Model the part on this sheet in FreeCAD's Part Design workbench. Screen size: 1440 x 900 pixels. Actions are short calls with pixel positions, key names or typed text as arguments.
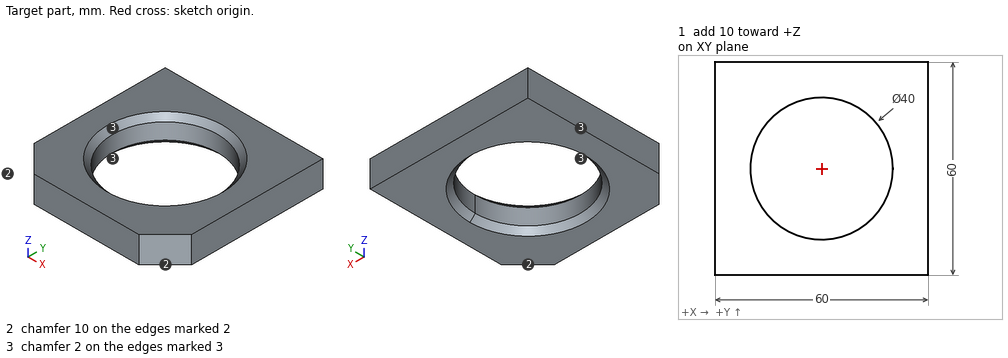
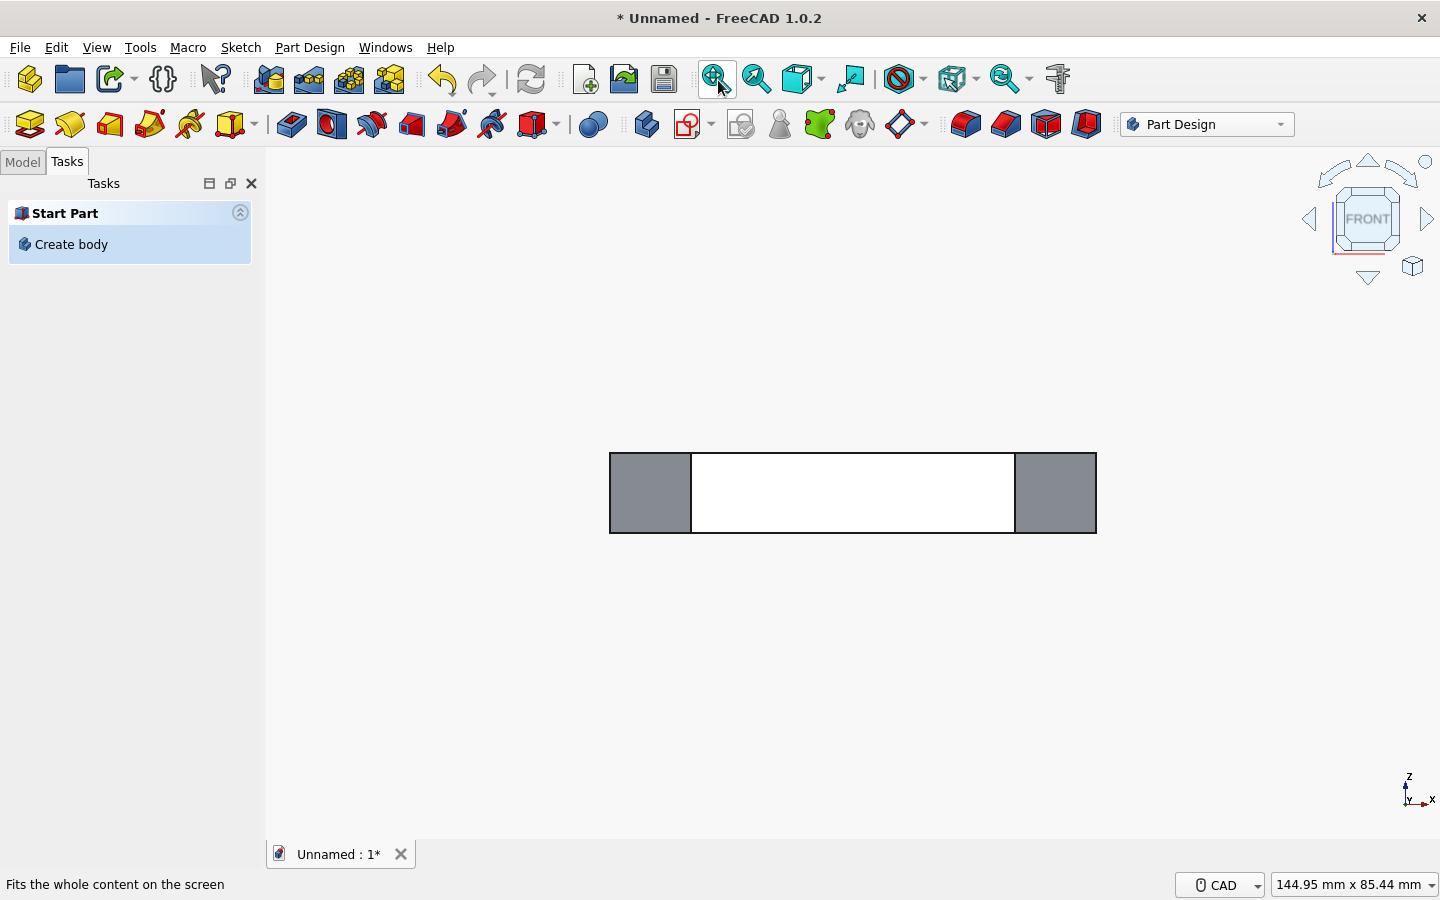
key(0)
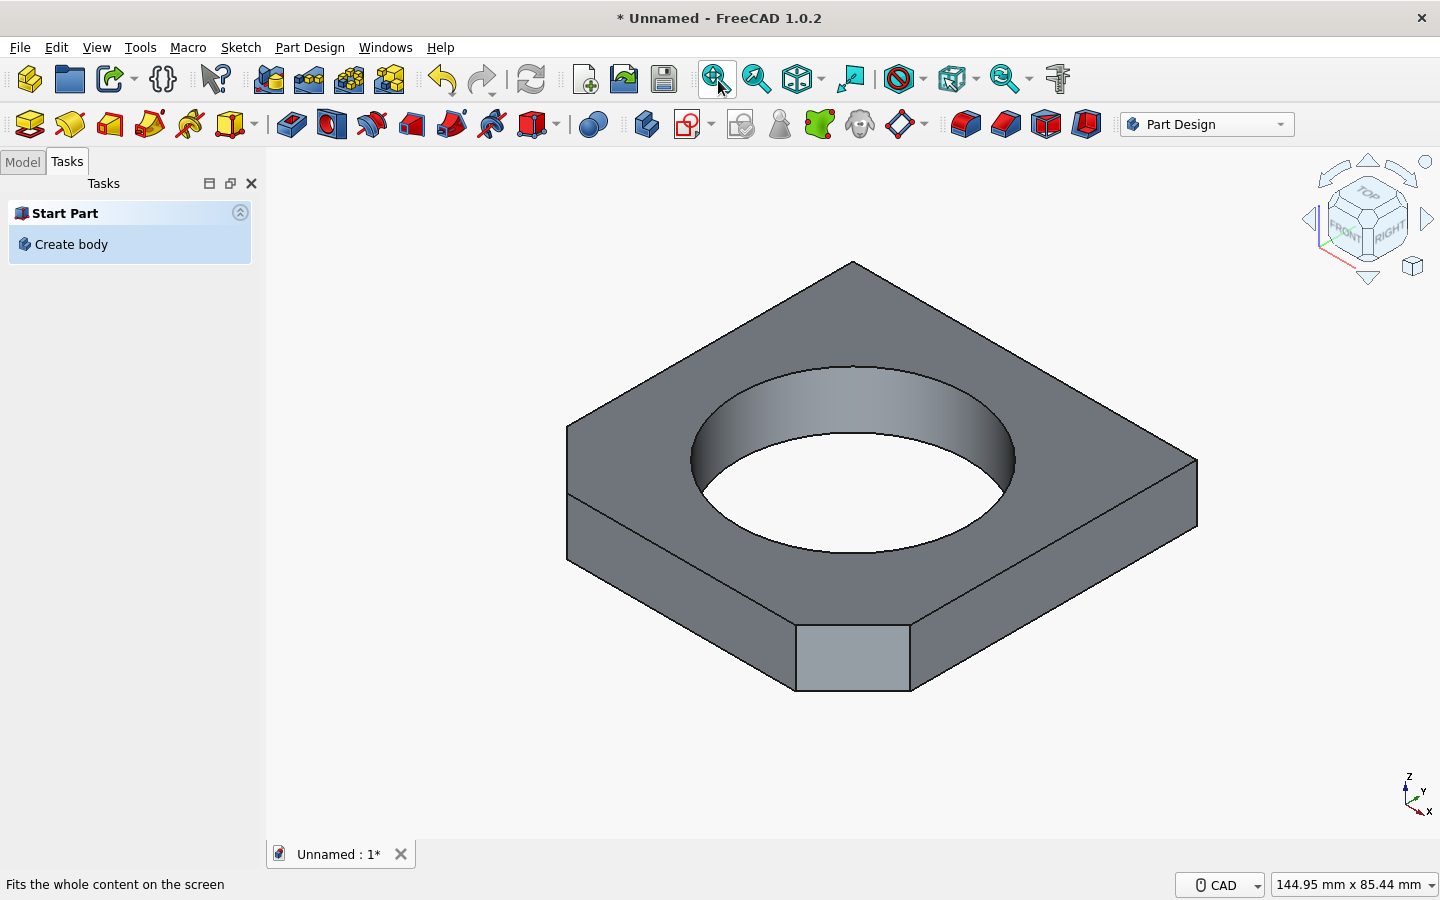
click(738, 393)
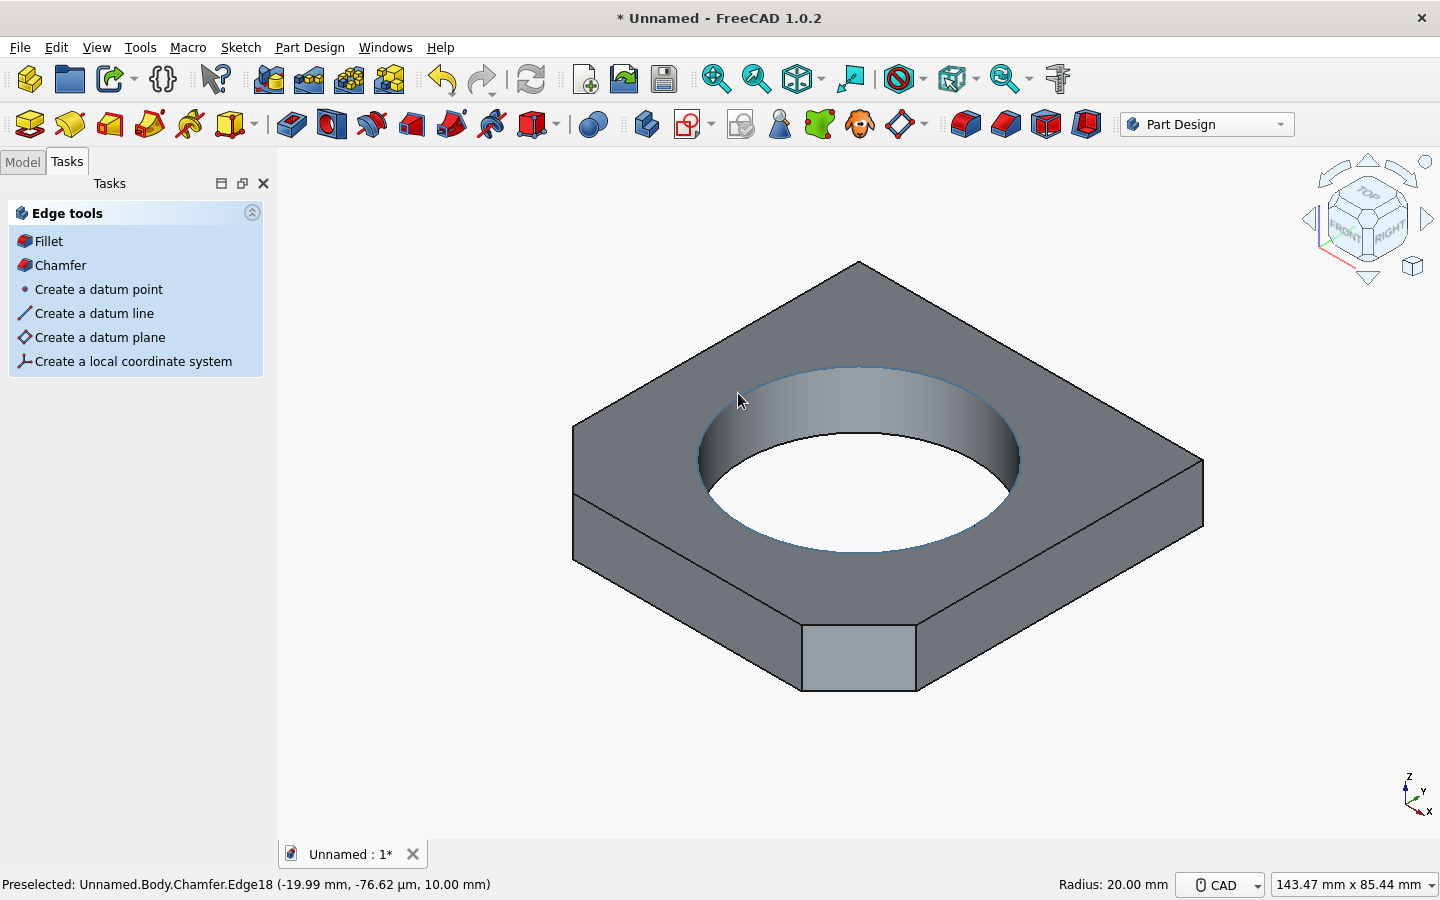
key(2)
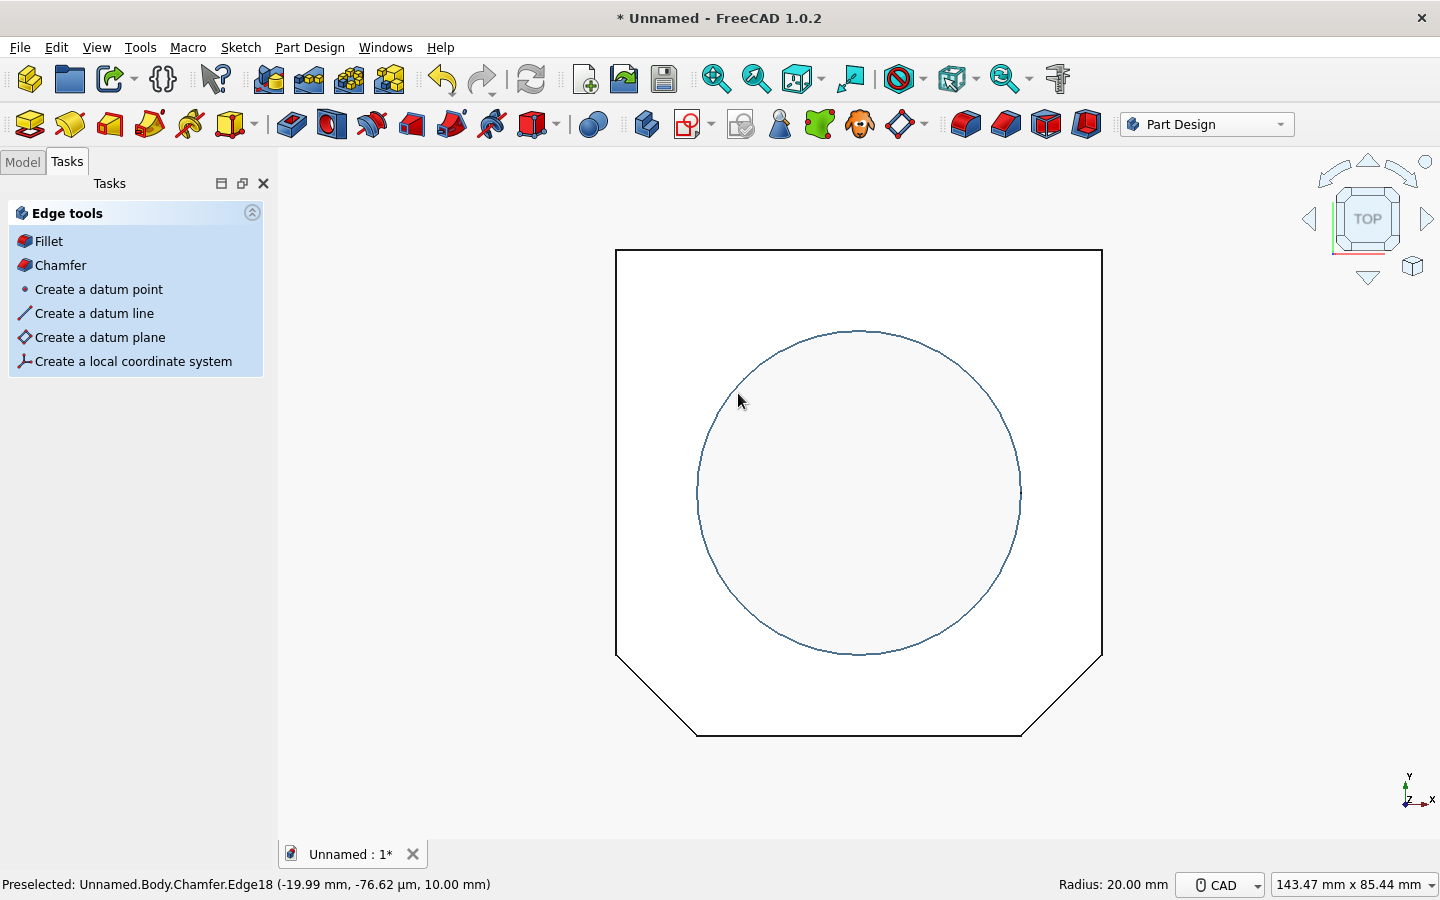
key(1)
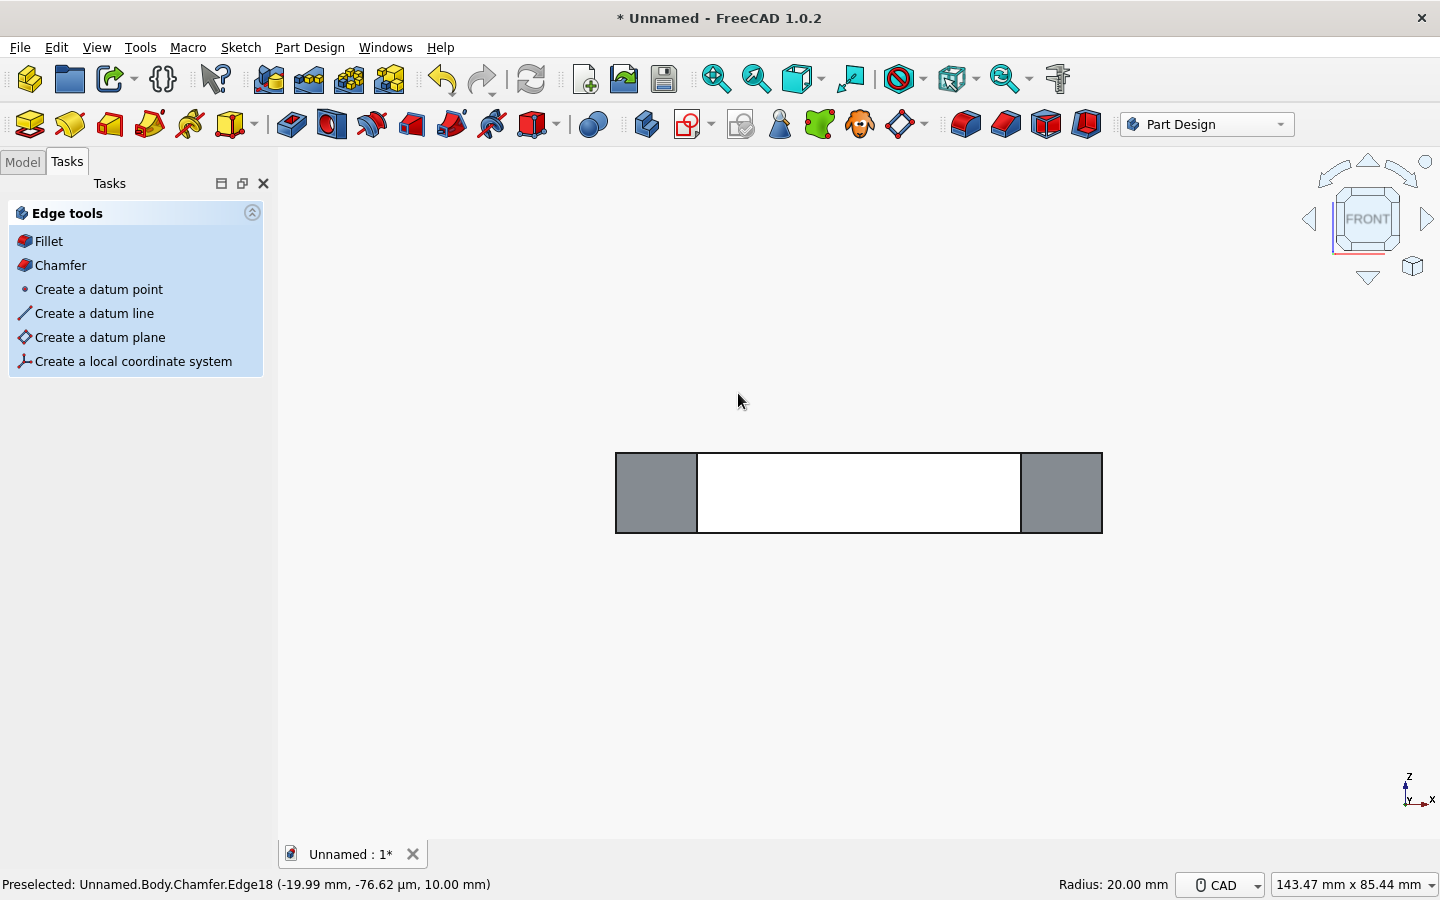
click(718, 80)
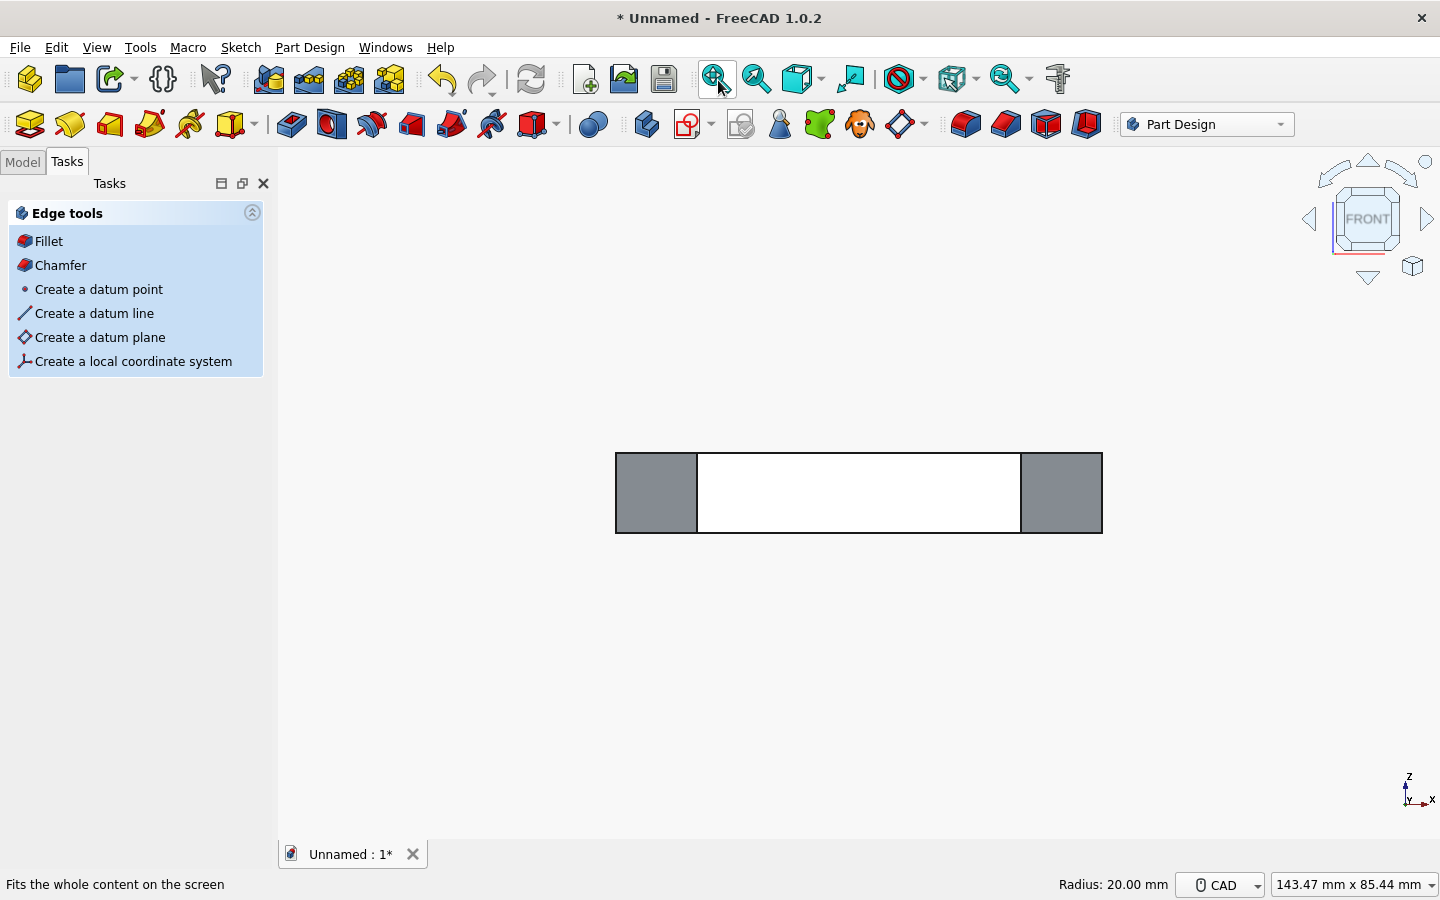
key(3)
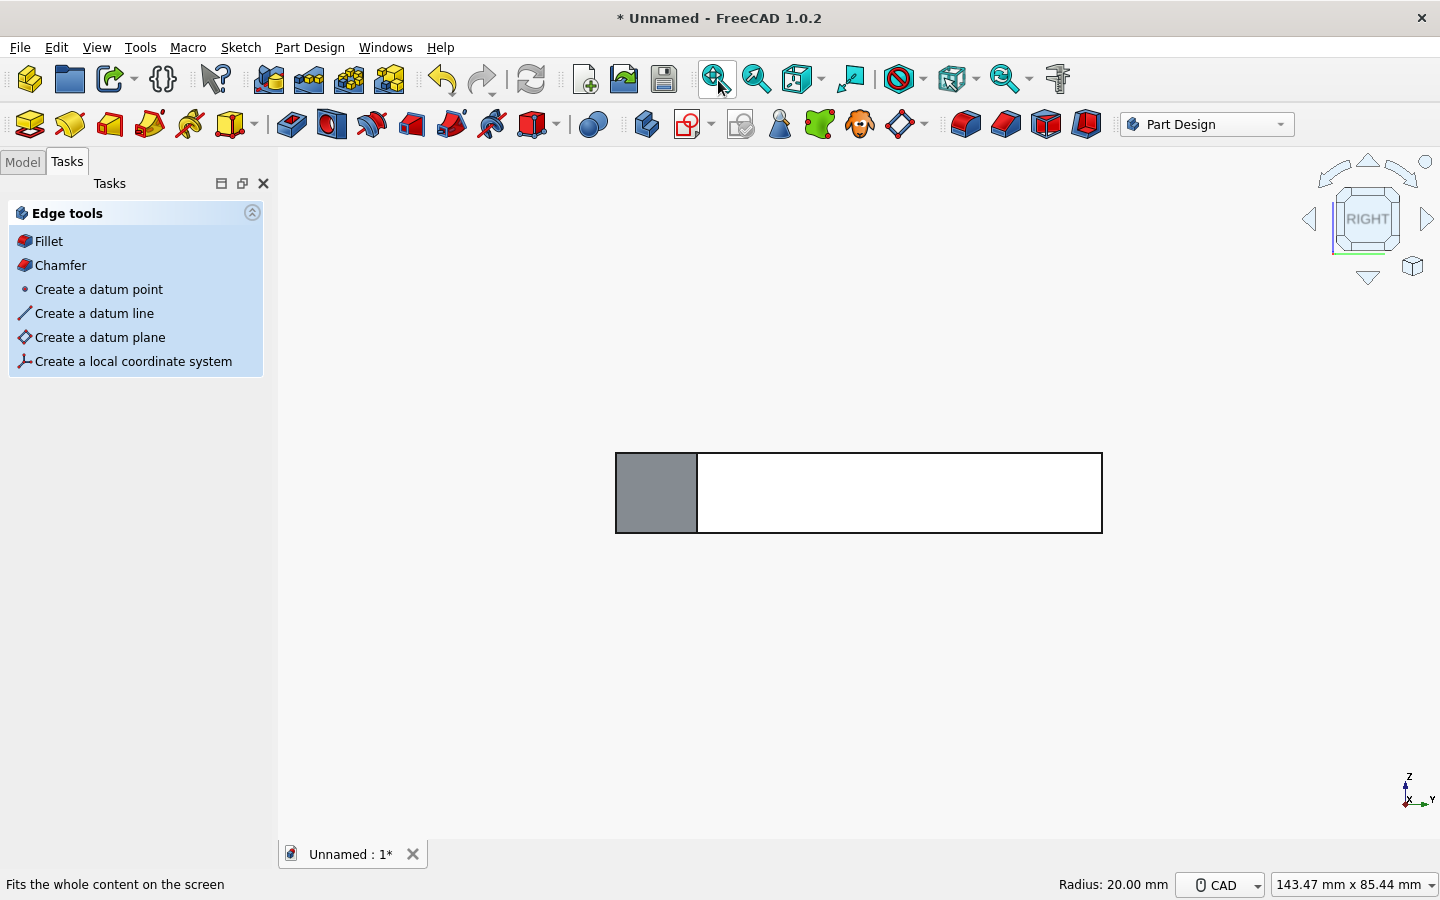
click(718, 80)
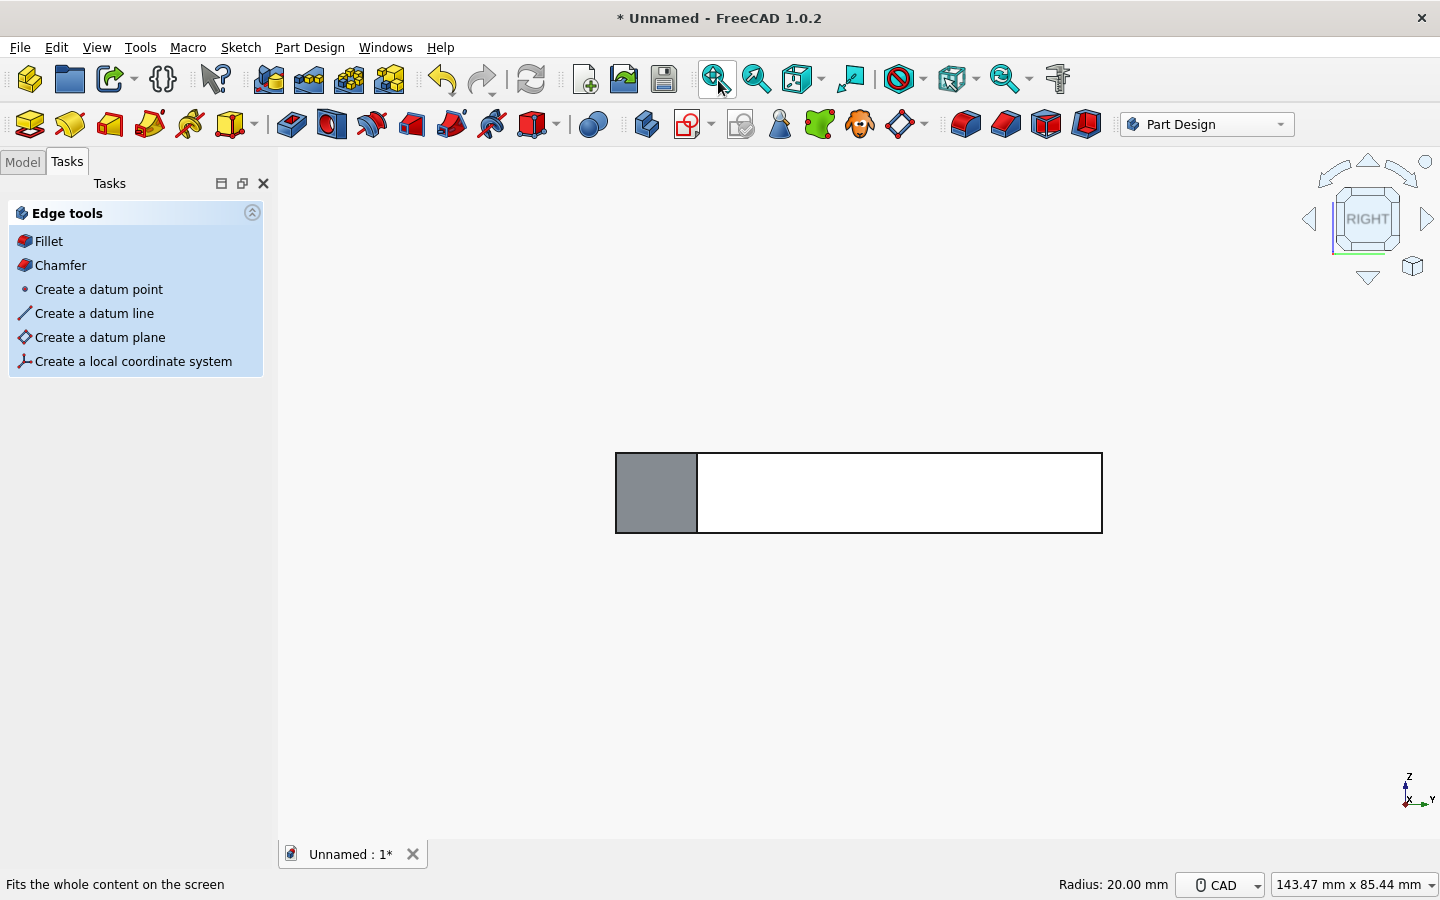
key(5)